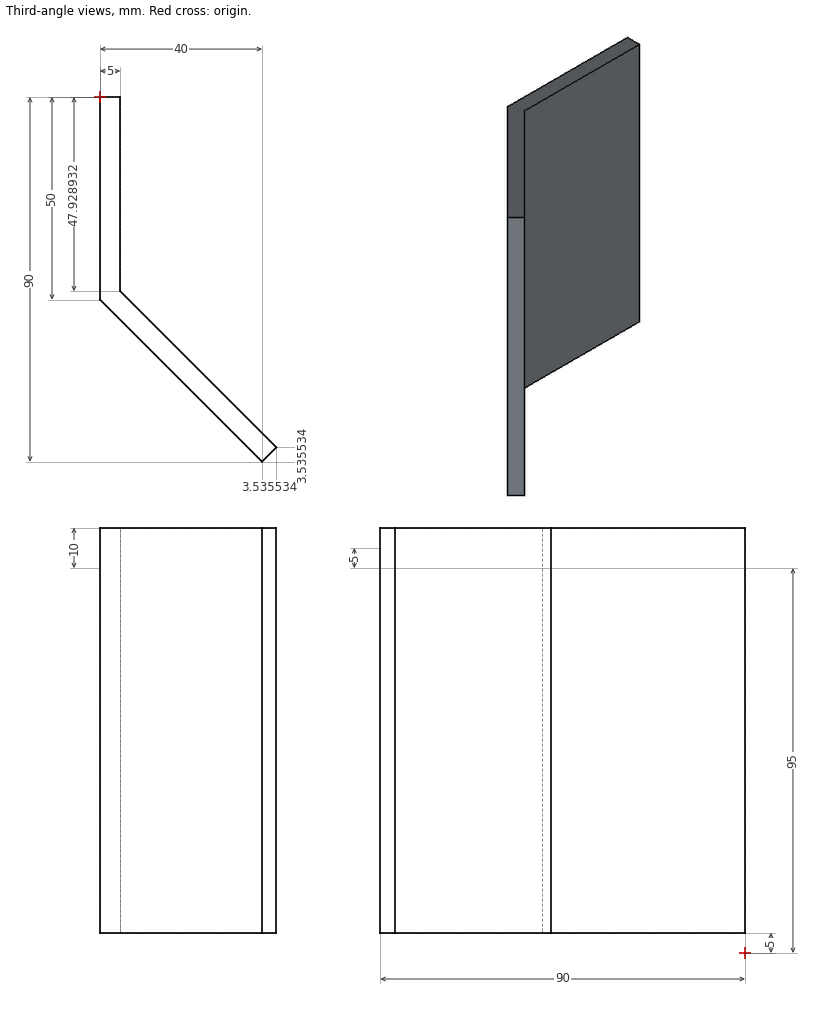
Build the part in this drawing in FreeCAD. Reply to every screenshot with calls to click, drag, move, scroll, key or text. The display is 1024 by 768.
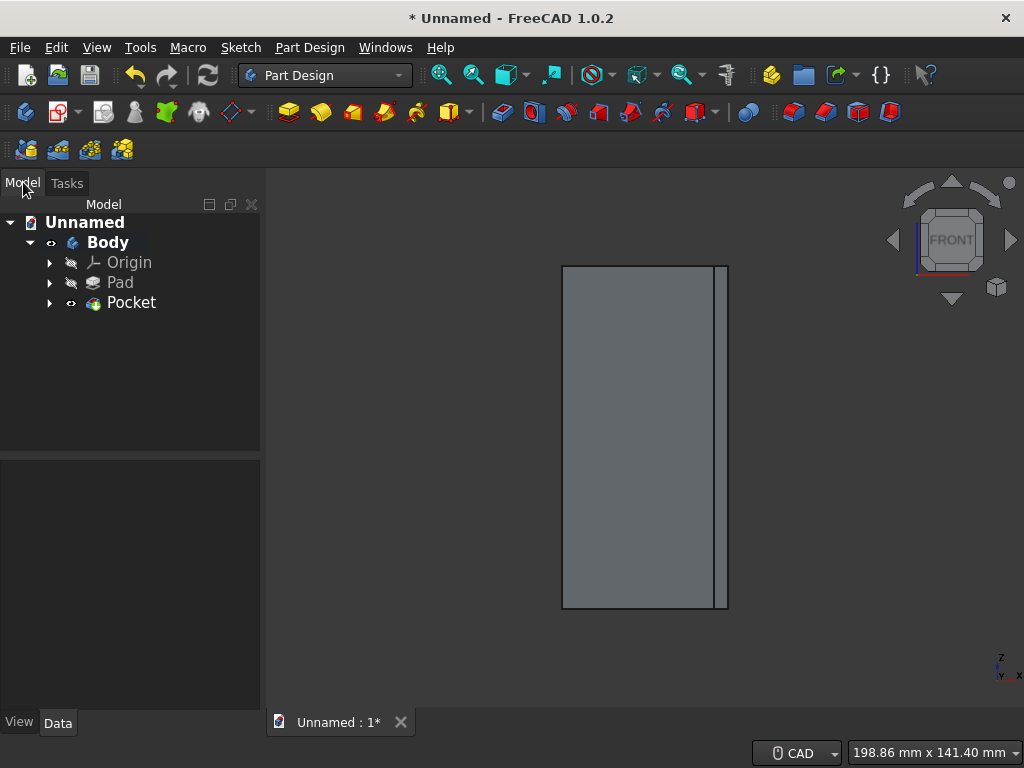
click(50, 263)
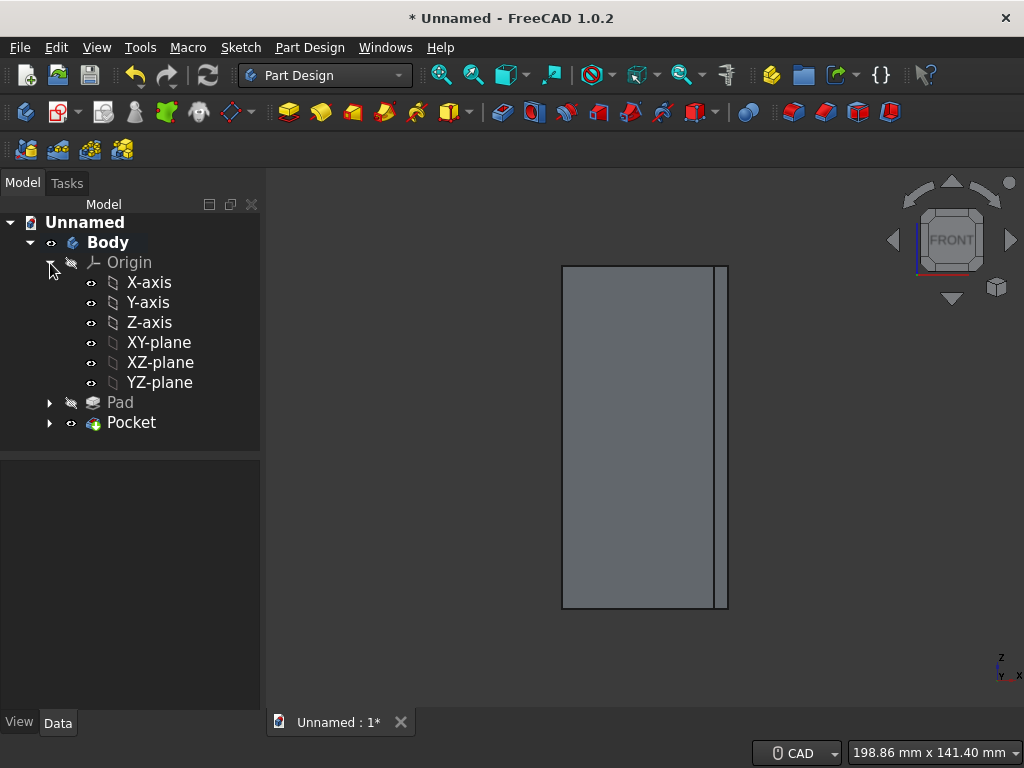
click(136, 343)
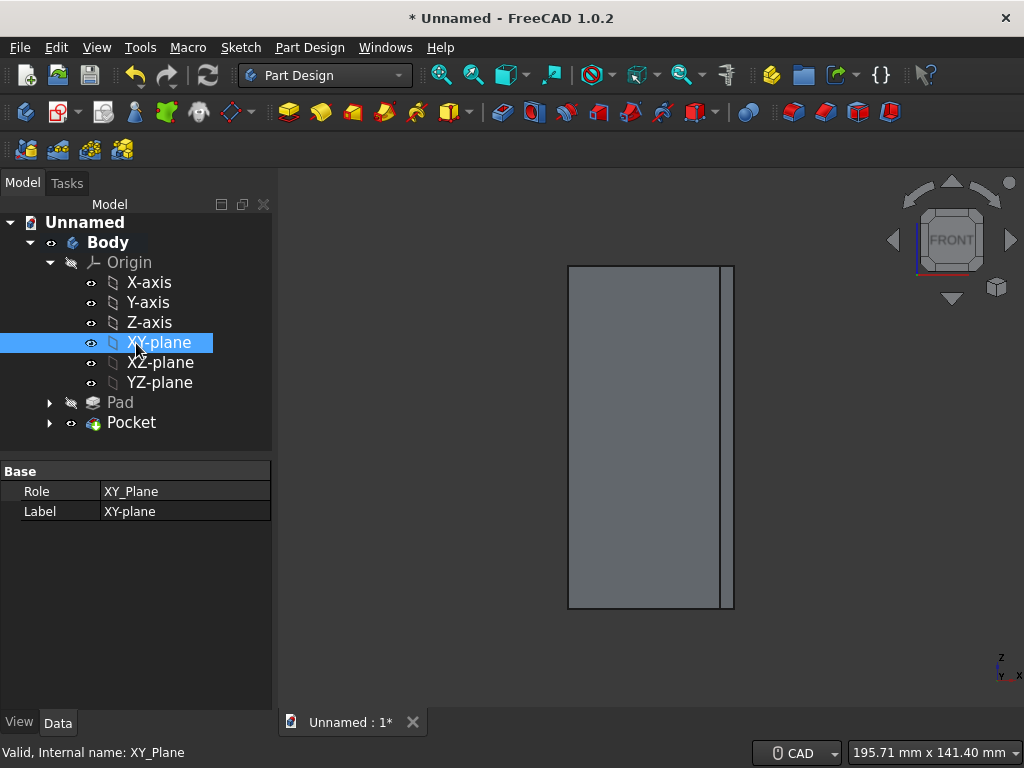
click(232, 112)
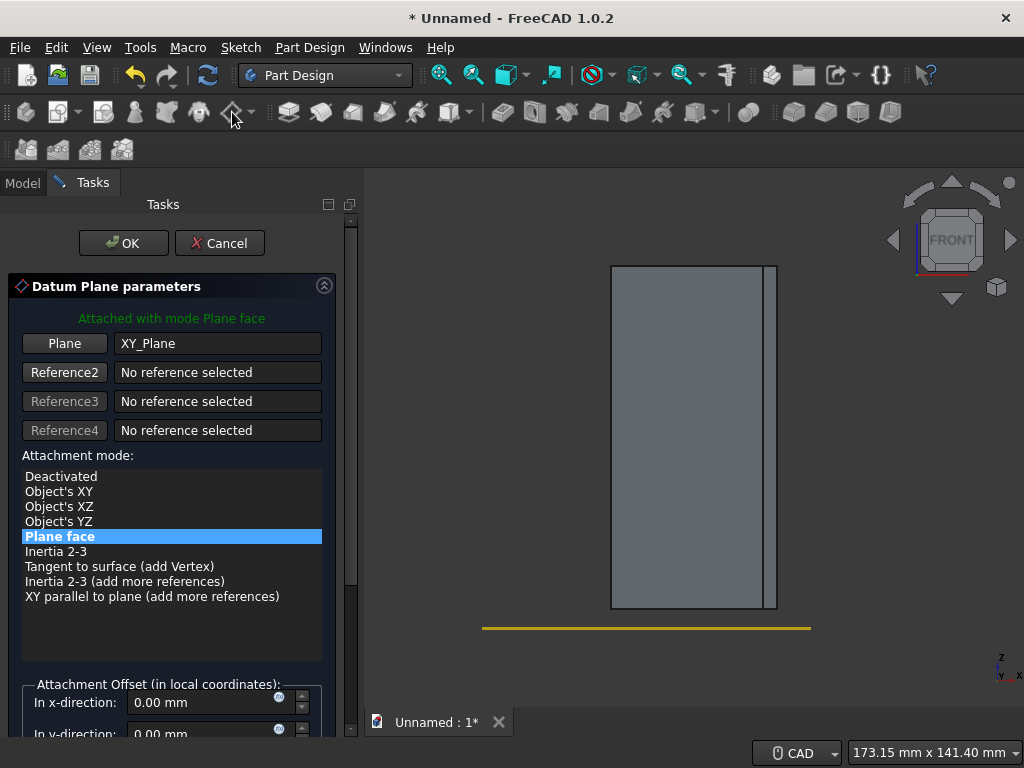
scroll(351, 475, down, 2)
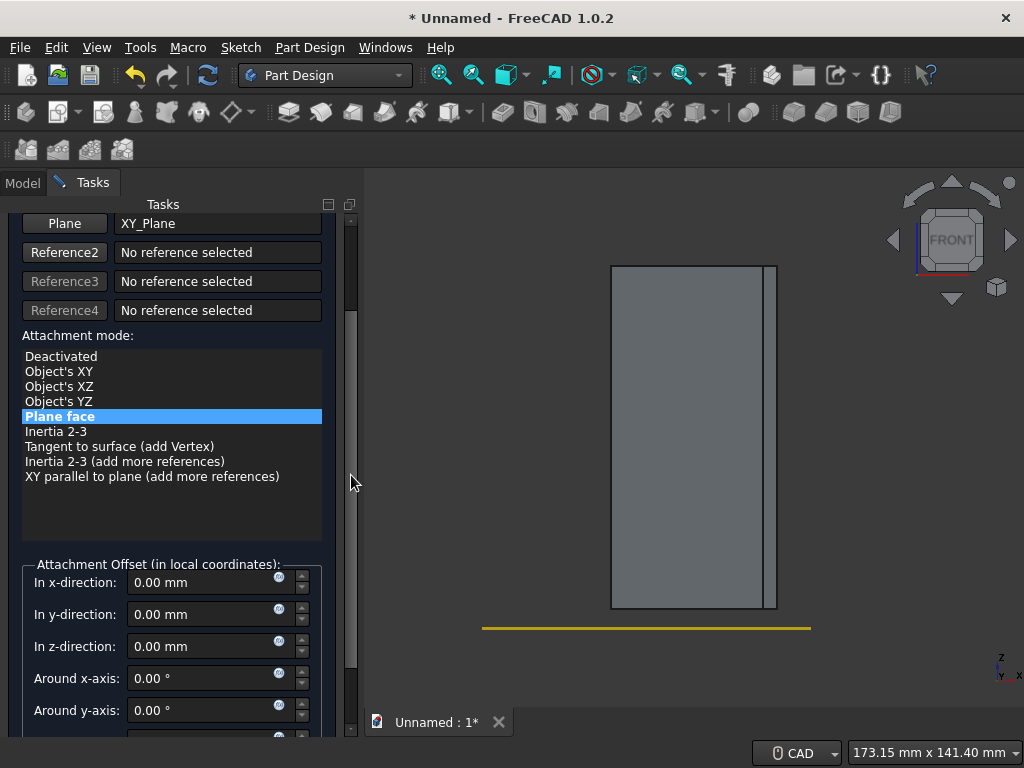
triple_click(210, 646)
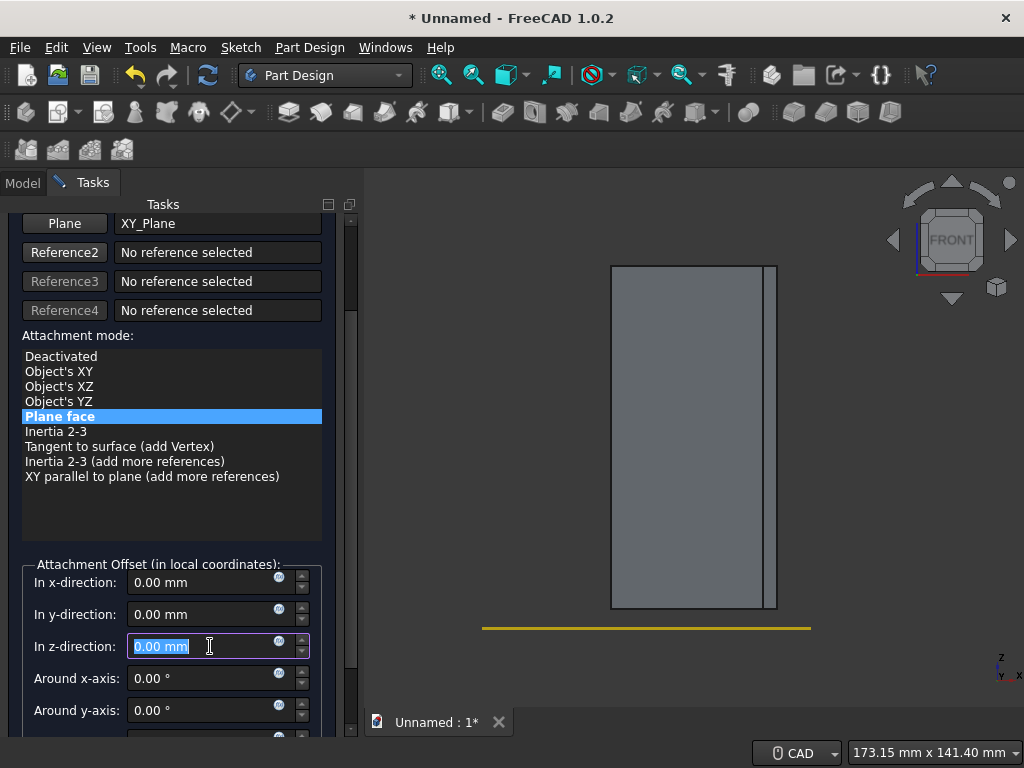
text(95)
key(Tab)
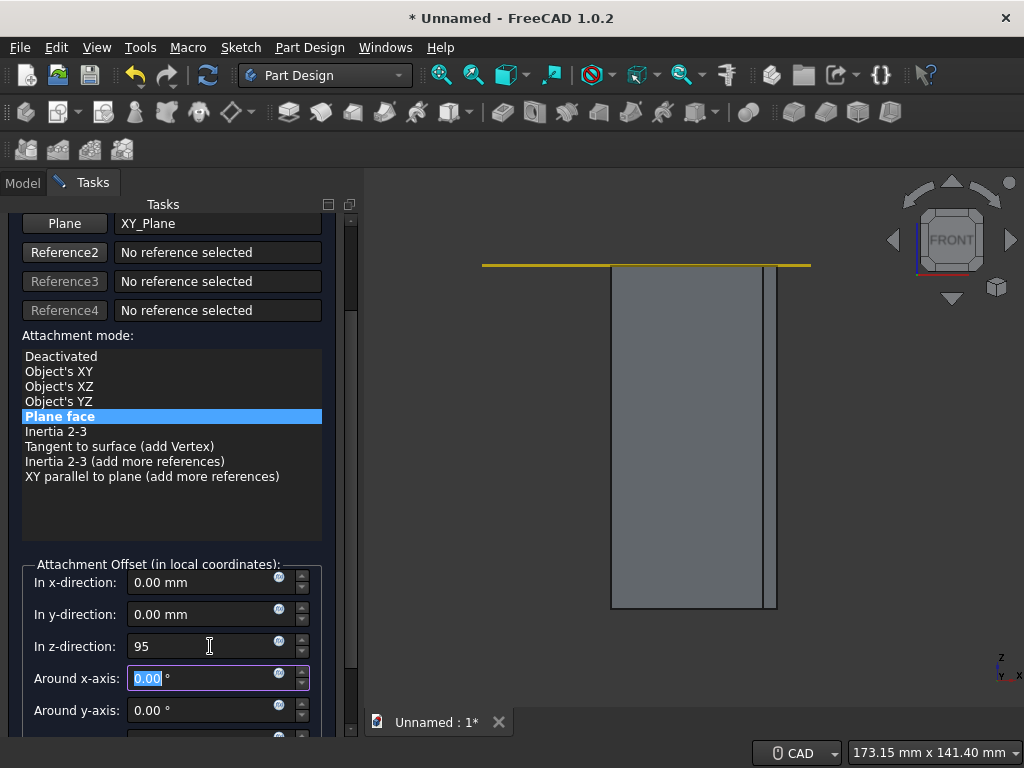
scroll(351, 475, up, 3)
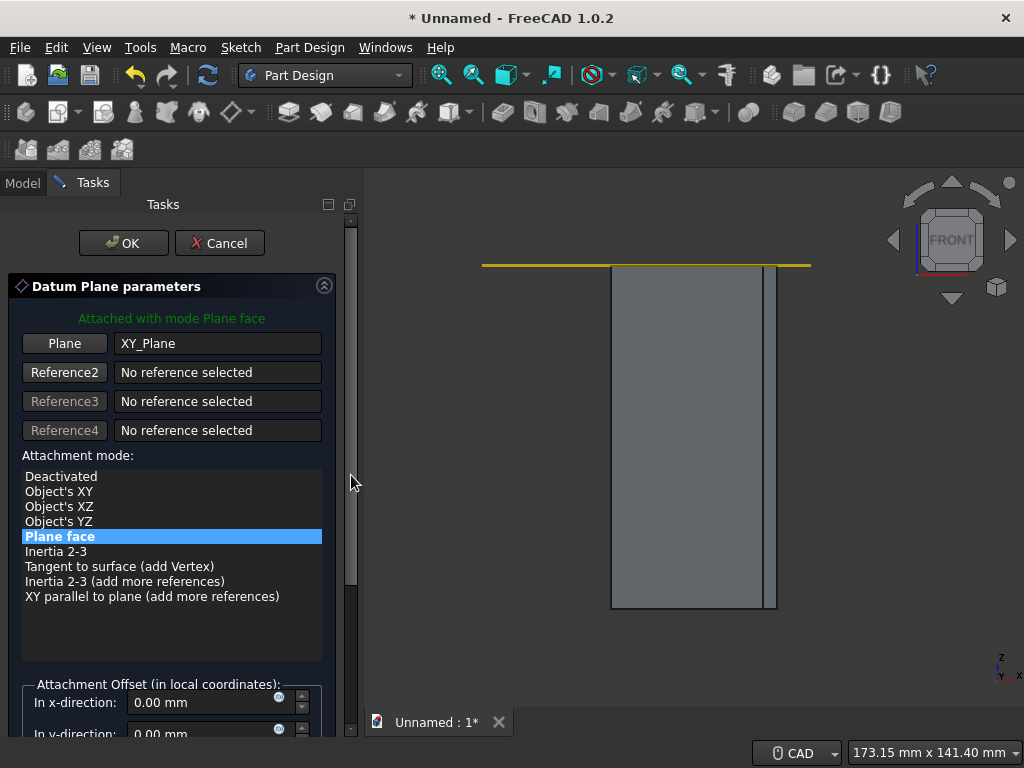
click(124, 243)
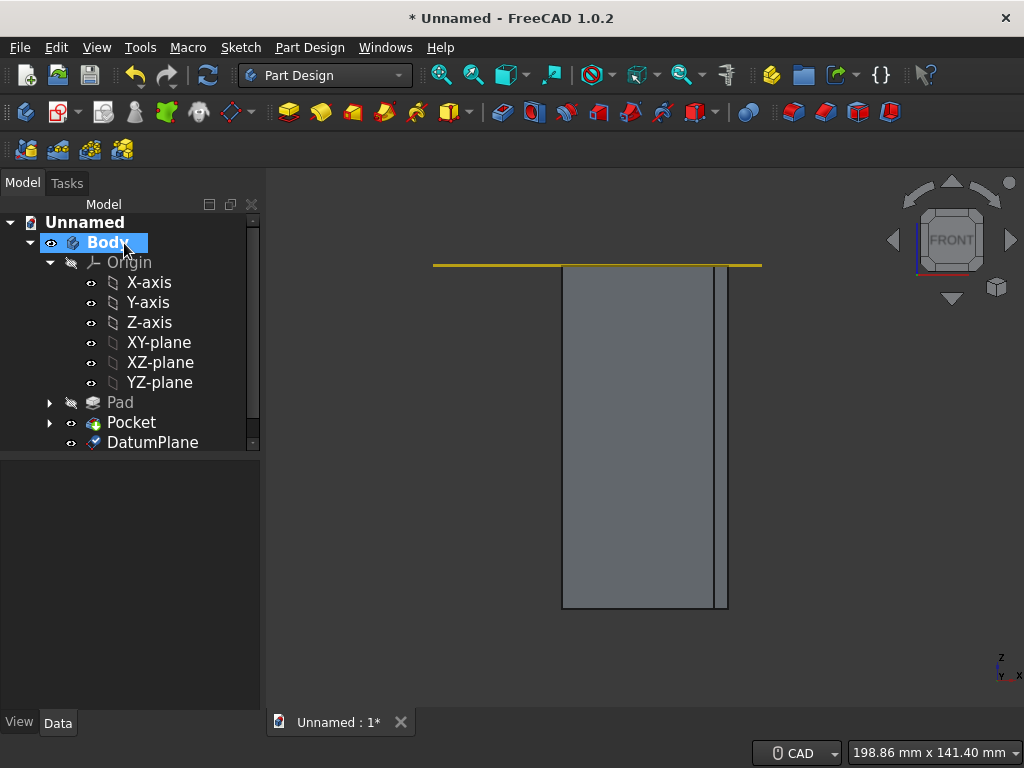
click(116, 443)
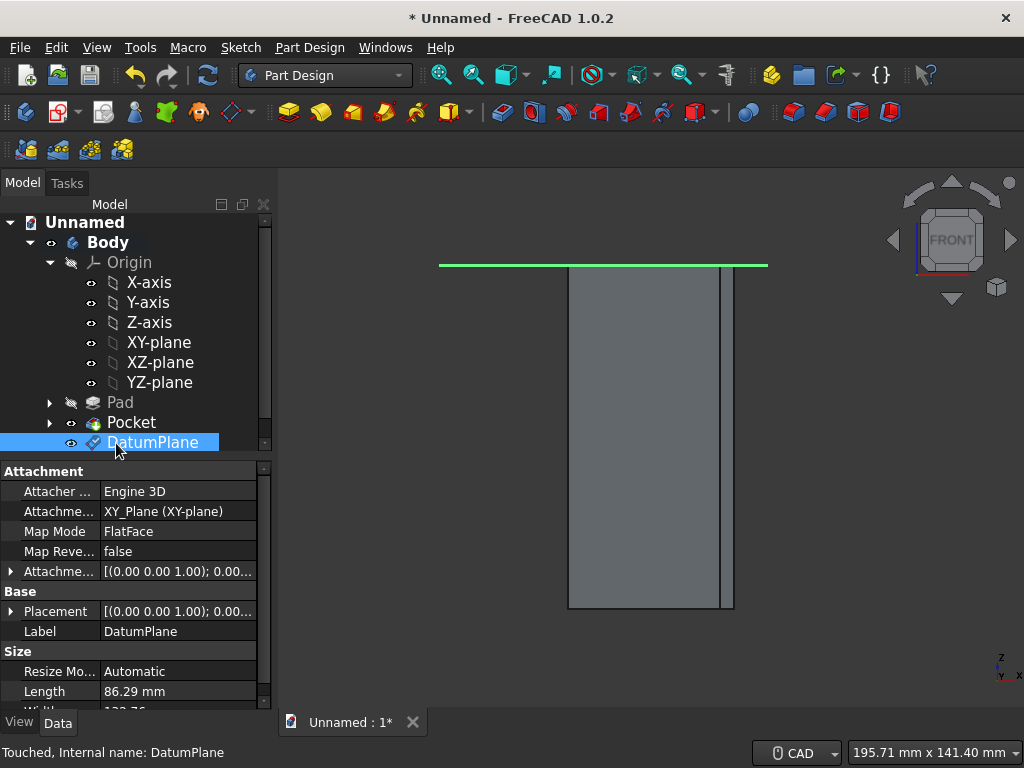
click(58, 112)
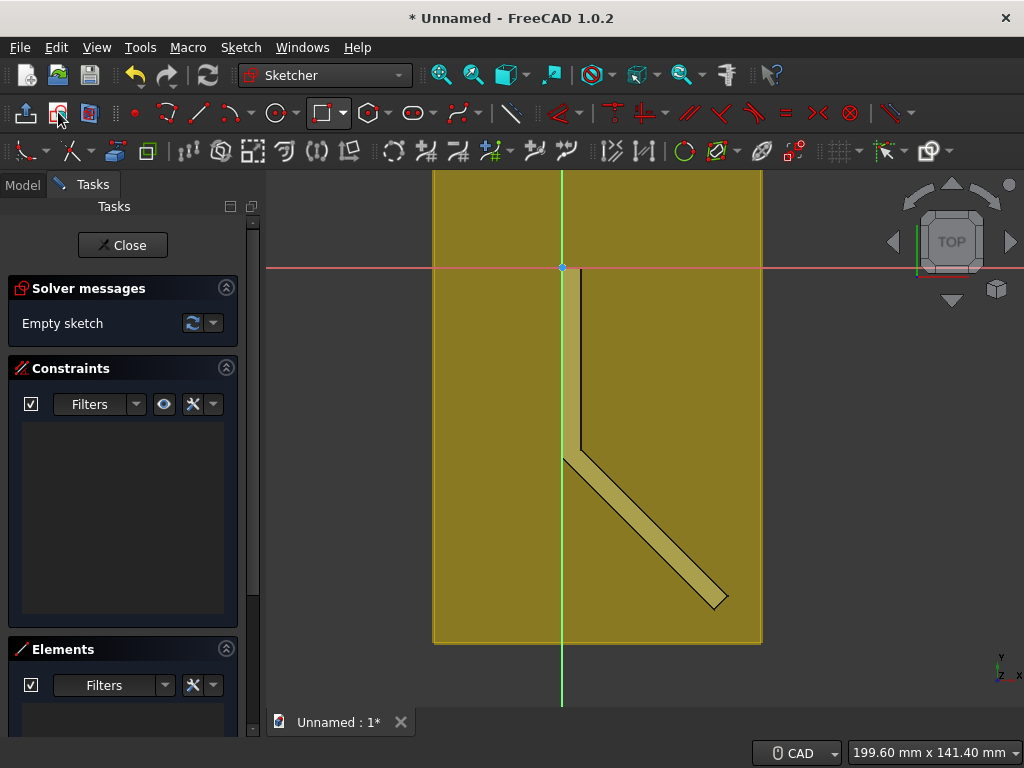
click(168, 114)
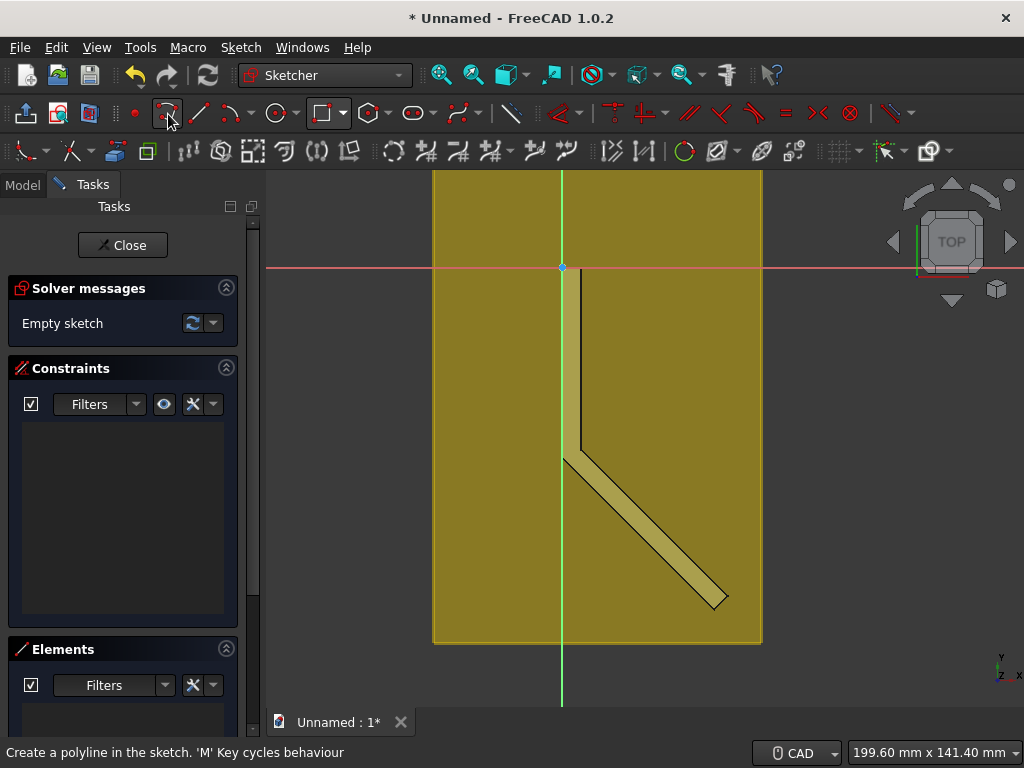
click(562, 268)
click(571, 457)
click(714, 609)
click(728, 596)
click(581, 450)
click(581, 277)
click(562, 268)
key(Escape)
key(Escape)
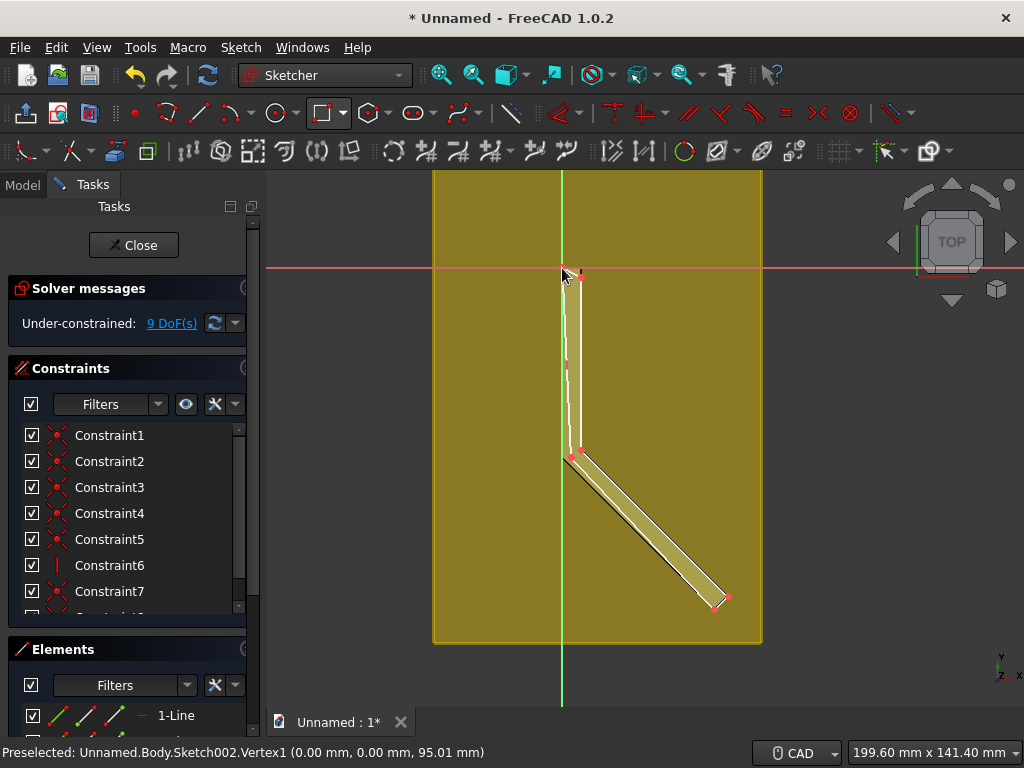
click(565, 325)